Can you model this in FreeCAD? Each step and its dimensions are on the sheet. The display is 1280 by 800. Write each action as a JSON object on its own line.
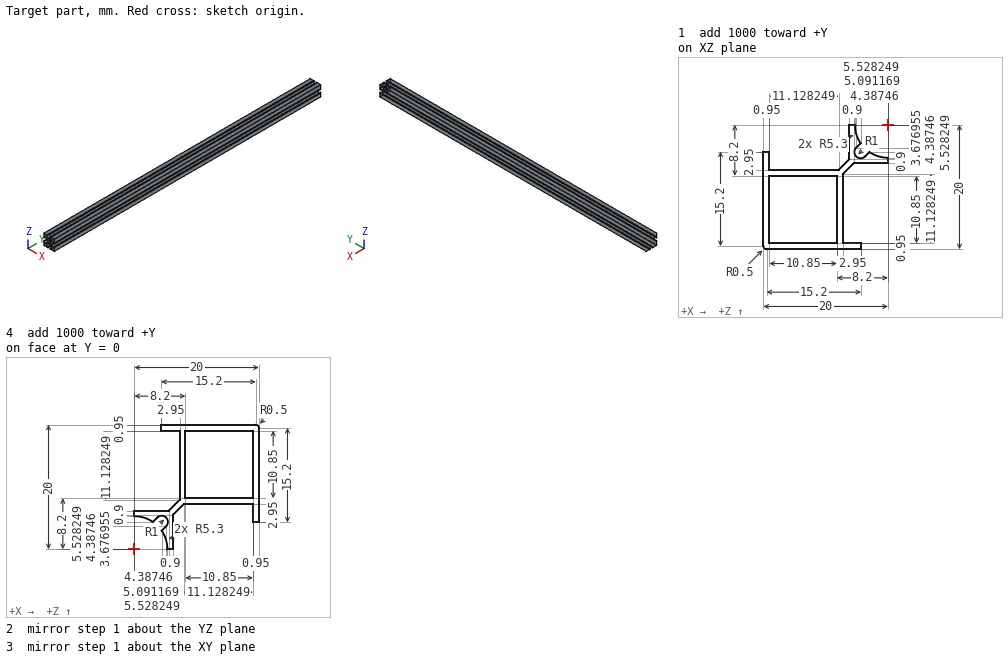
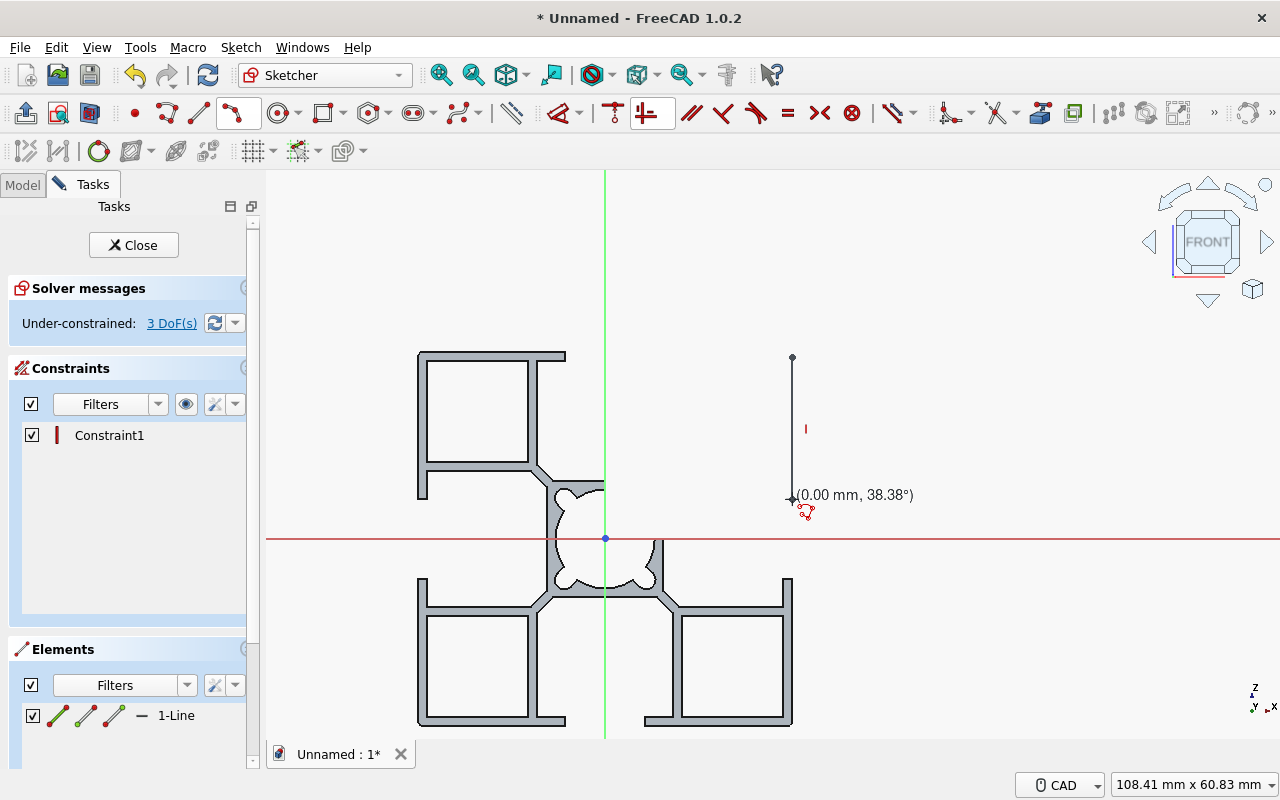
{"action": "scroll", "coordinate": [783, 499], "scroll_direction": "up", "scroll_amount": 3}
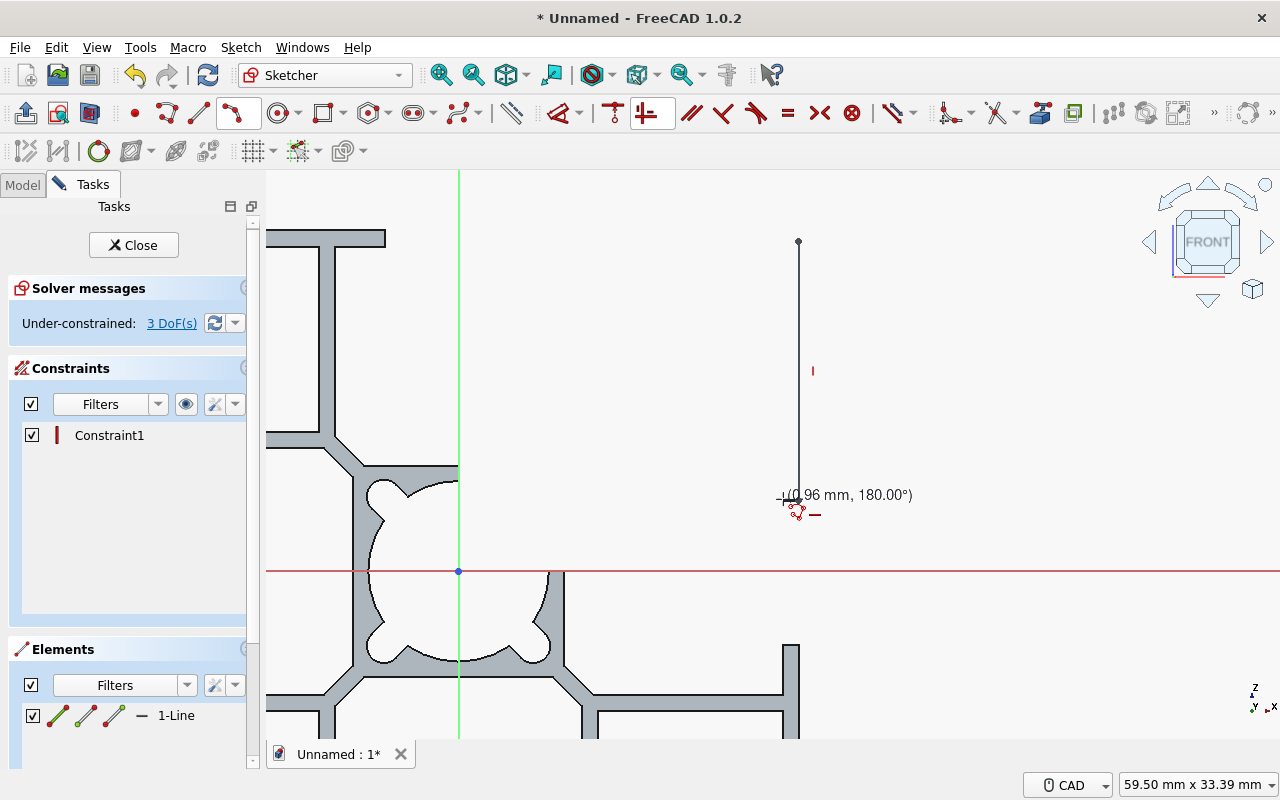
{"action": "left_click", "coordinate": [783, 499]}
{"action": "left_click", "coordinate": [783, 448]}
{"action": "left_click", "coordinate": [594, 448]}
{"action": "left_click", "coordinate": [564, 477]}
{"action": "left_click", "coordinate": [564, 571]}
{"action": "left_click", "coordinate": [549, 562]}
{"action": "right_click", "coordinate": [549, 562]}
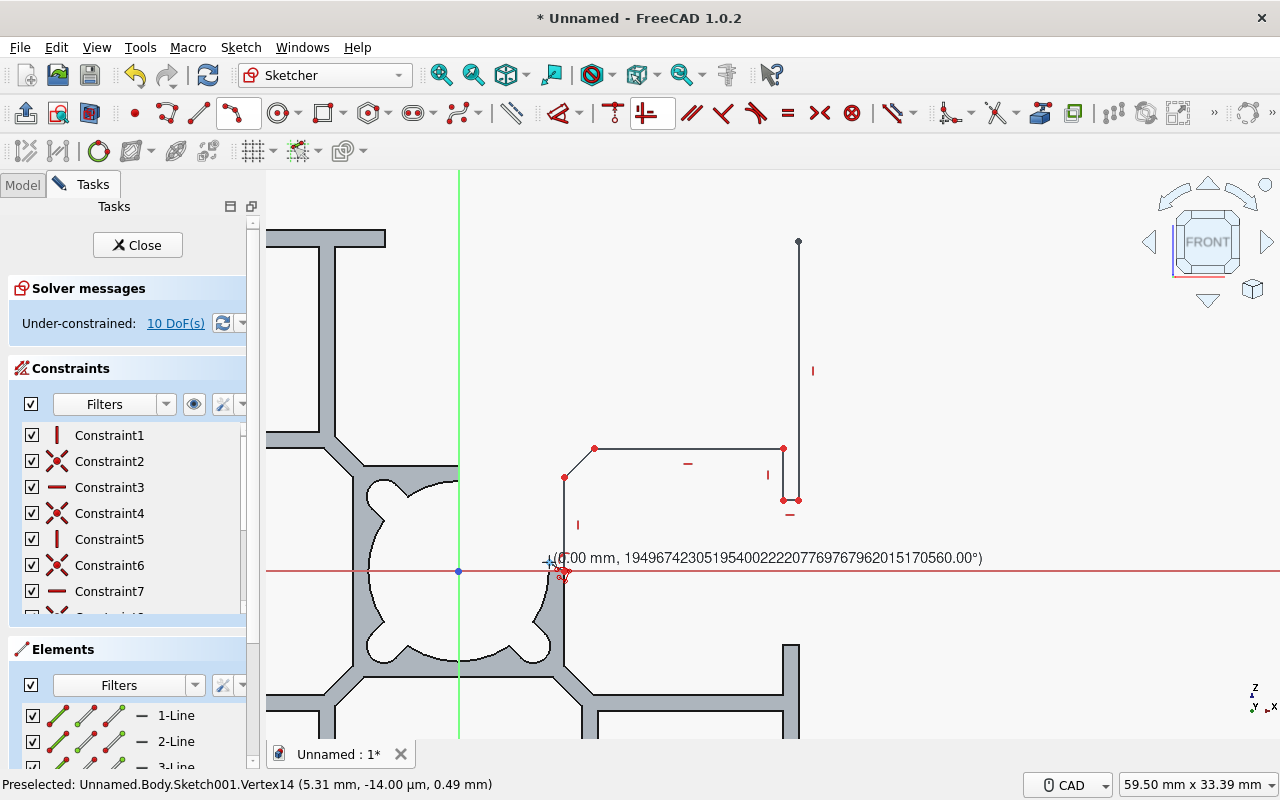
{"action": "key", "text": "g l"}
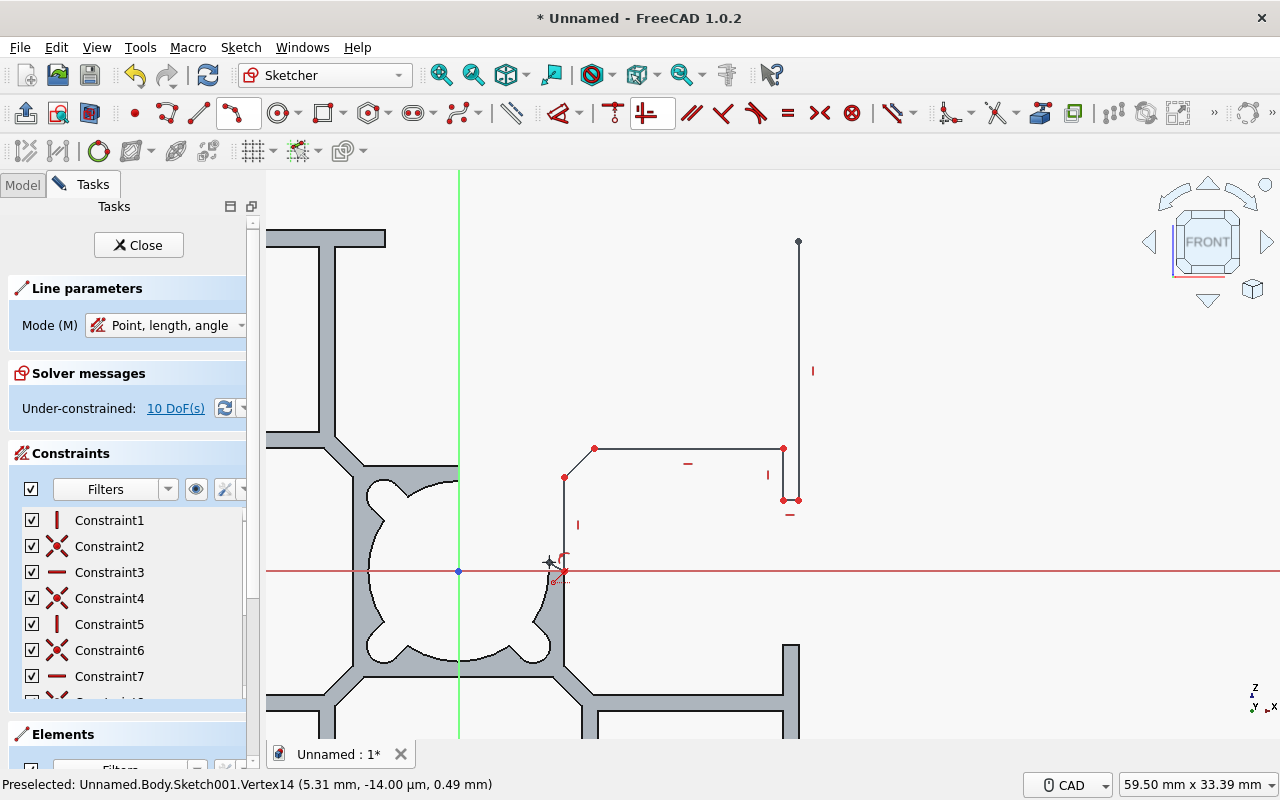
{"action": "left_click", "coordinate": [533, 521]}
{"action": "left_click", "coordinate": [545, 509]}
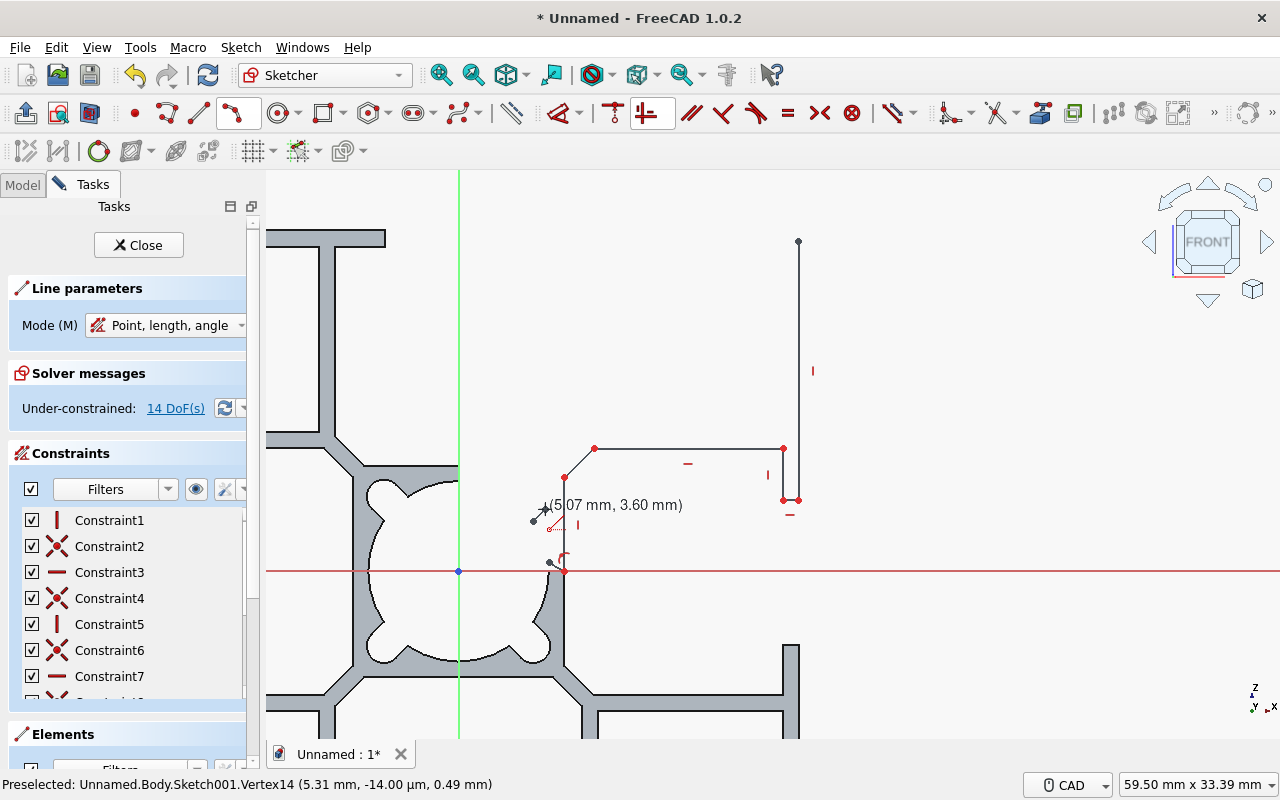
{"action": "left_click", "coordinate": [521, 485]}
{"action": "left_click", "coordinate": [509, 497]}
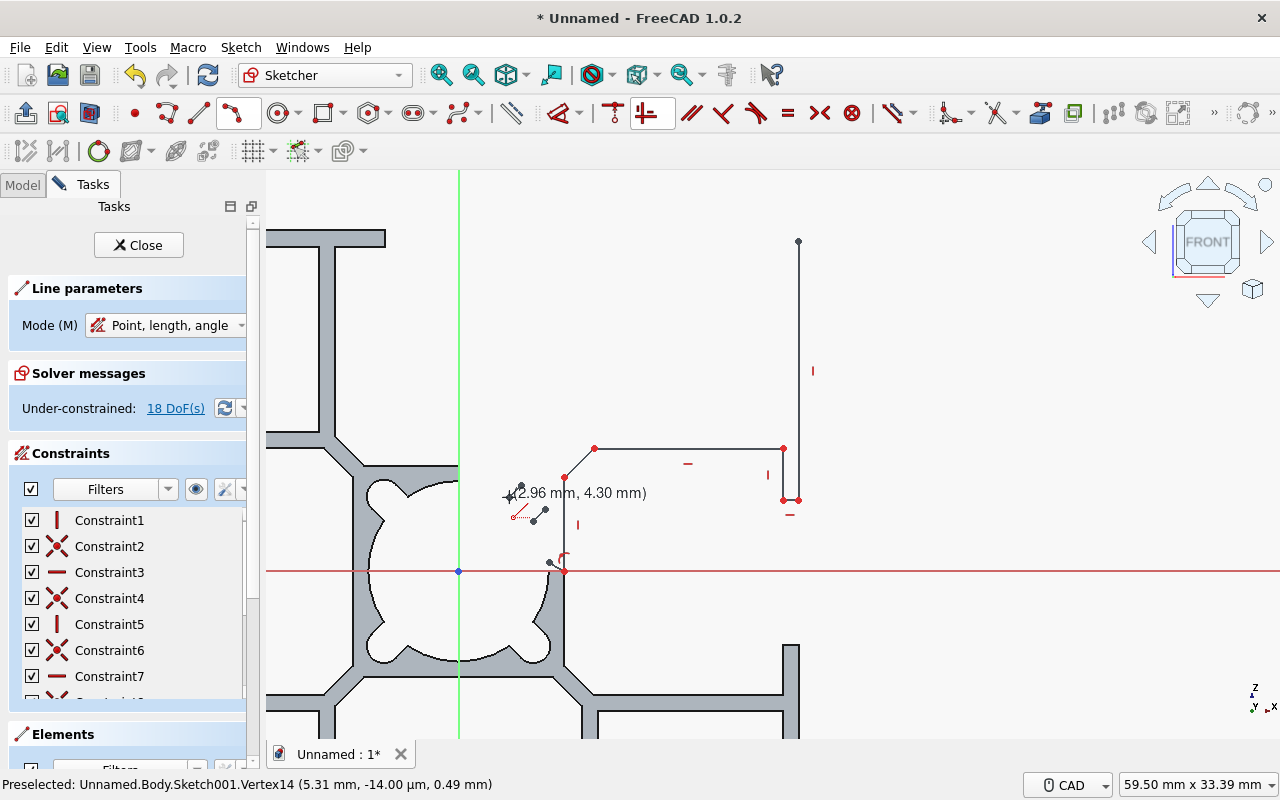
{"action": "left_click", "coordinate": [168, 114]}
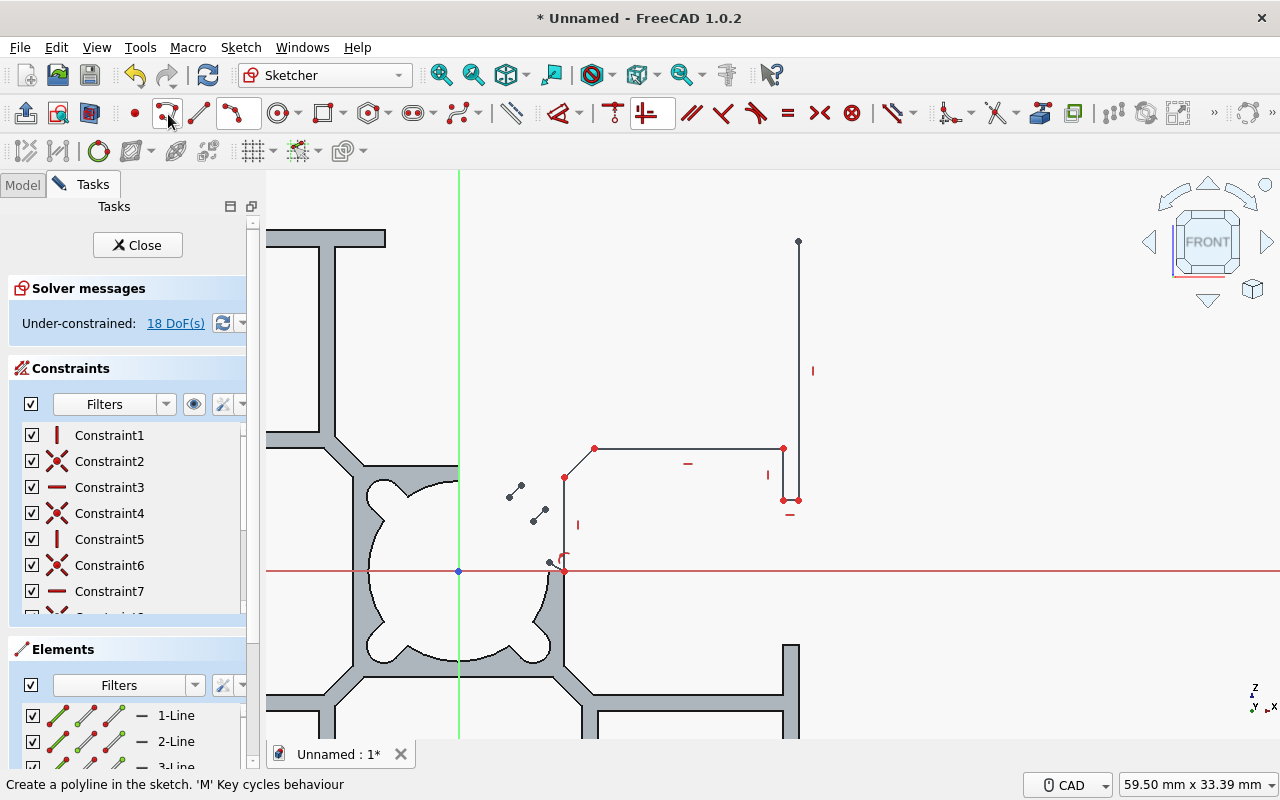
{"action": "left_click", "coordinate": [459, 481]}
{"action": "left_click", "coordinate": [468, 466]}
{"action": "left_click", "coordinate": [553, 466]}
{"action": "left_click", "coordinate": [582, 436]}
{"action": "left_click", "coordinate": [582, 247]}
{"action": "left_click", "coordinate": [532, 247]}
{"action": "left_click", "coordinate": [532, 230]}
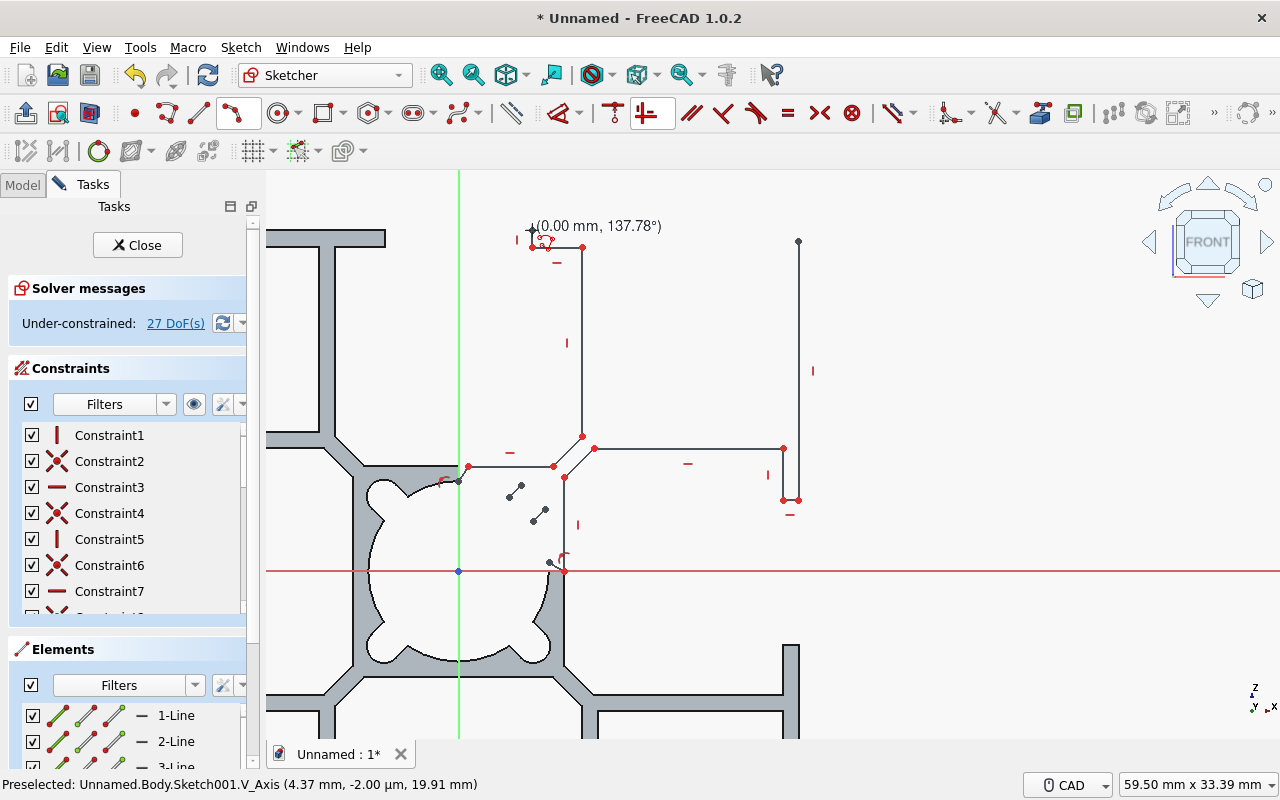
{"action": "scroll", "coordinate": [791, 230], "scroll_direction": "up", "scroll_amount": 2}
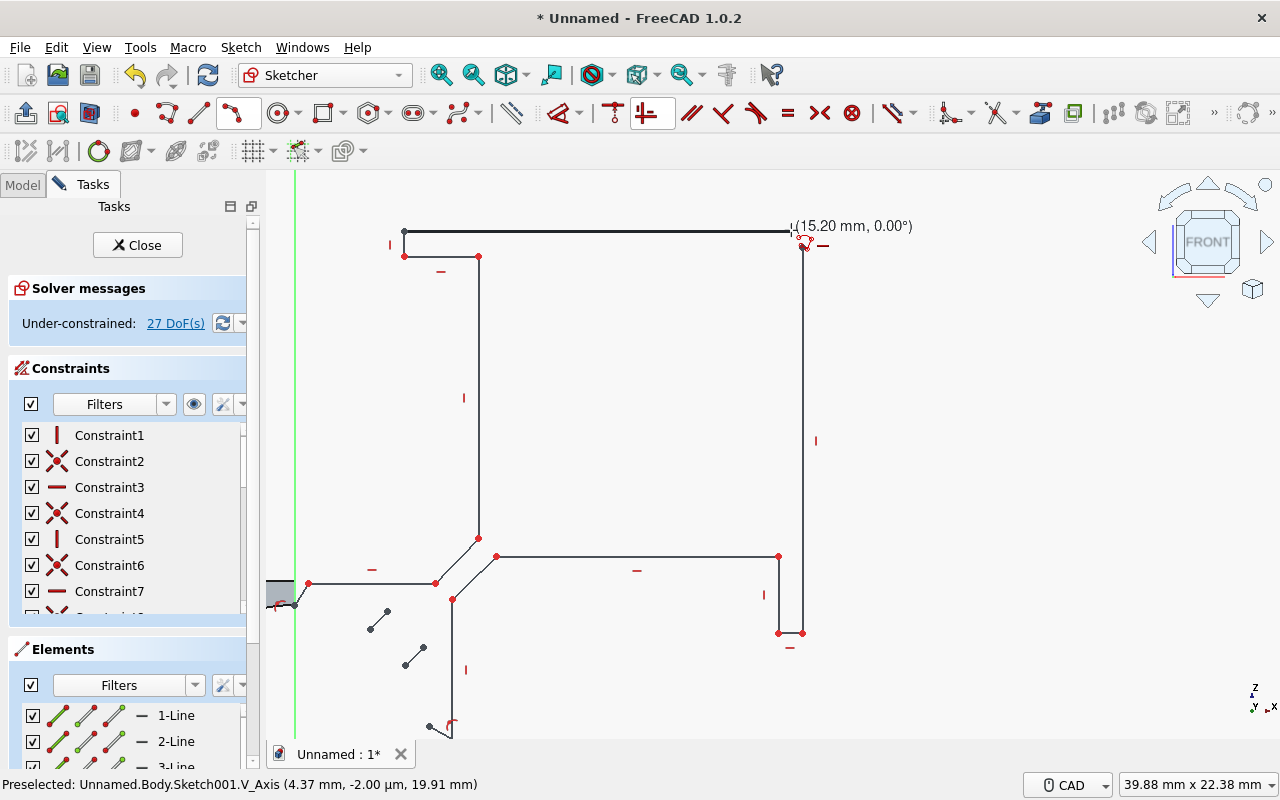
{"action": "left_click", "coordinate": [791, 230]}
{"action": "right_click", "coordinate": [791, 230]}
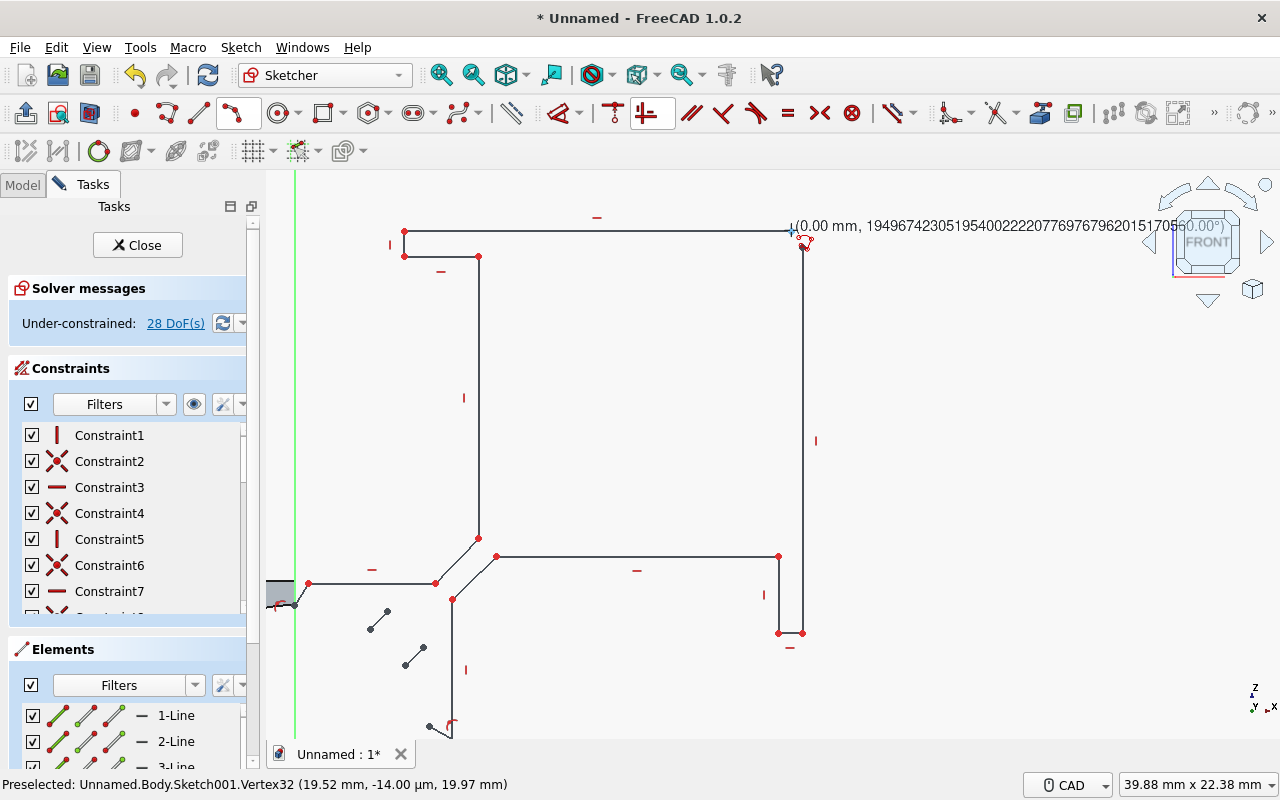
{"action": "key", "text": "g 3 a"}